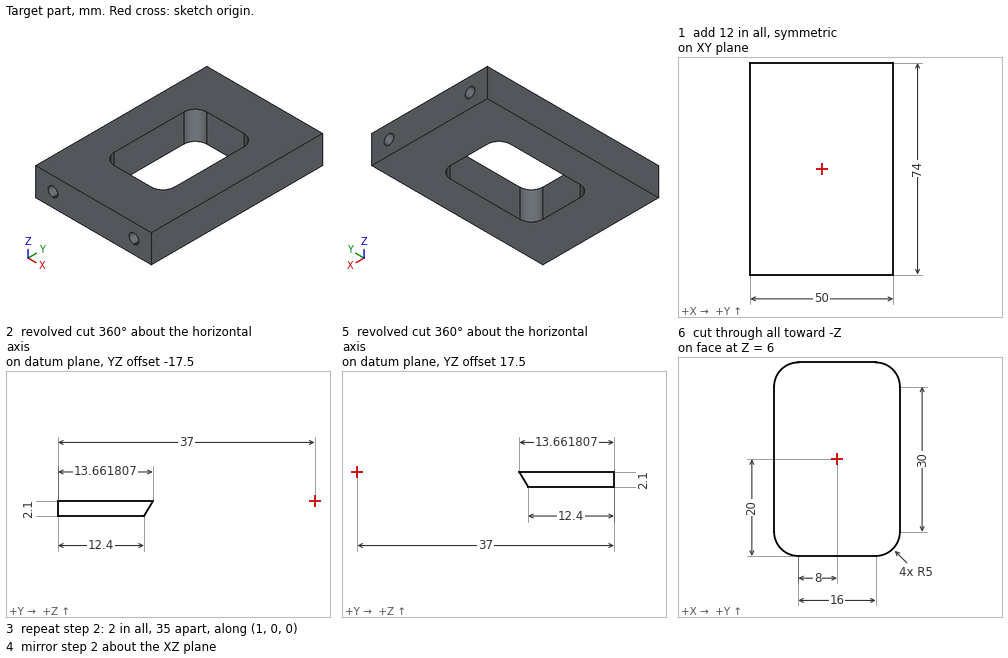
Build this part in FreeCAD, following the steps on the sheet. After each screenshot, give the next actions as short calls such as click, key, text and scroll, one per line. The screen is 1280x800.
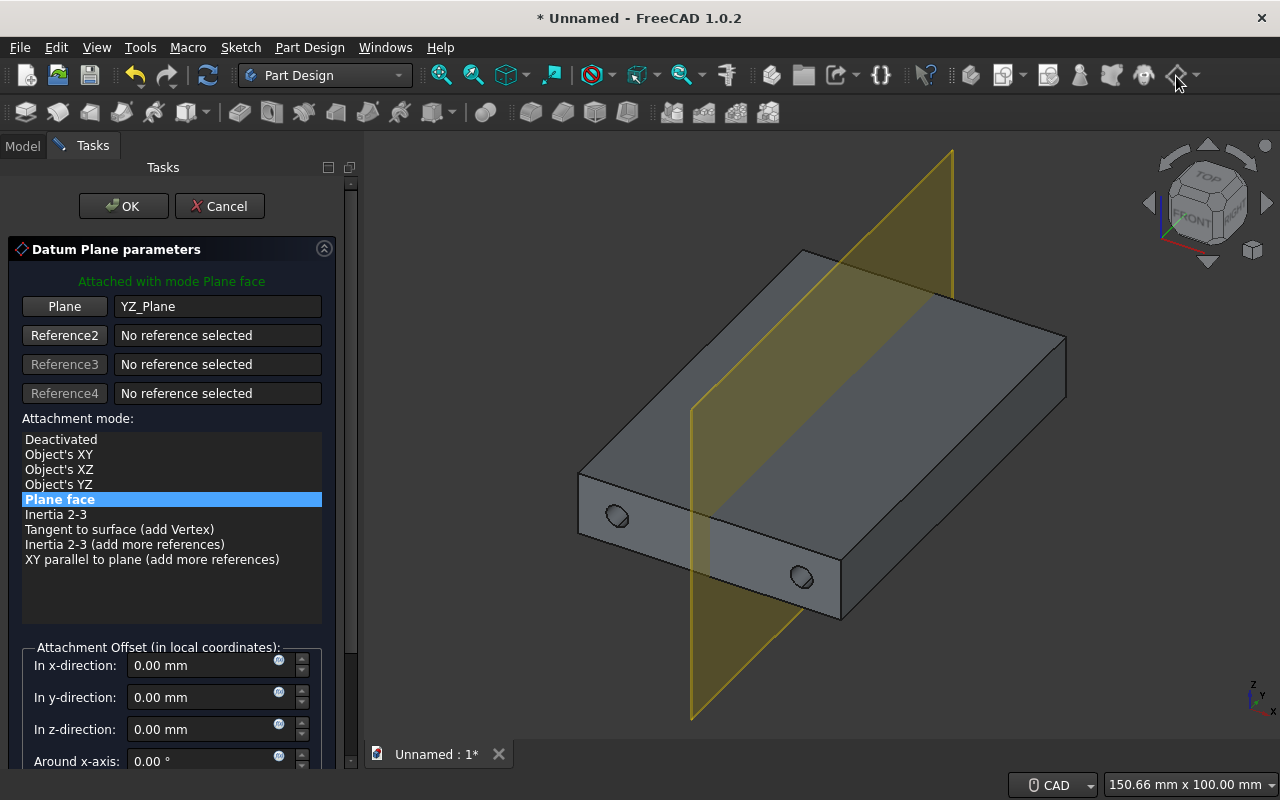
triple_click(210, 729)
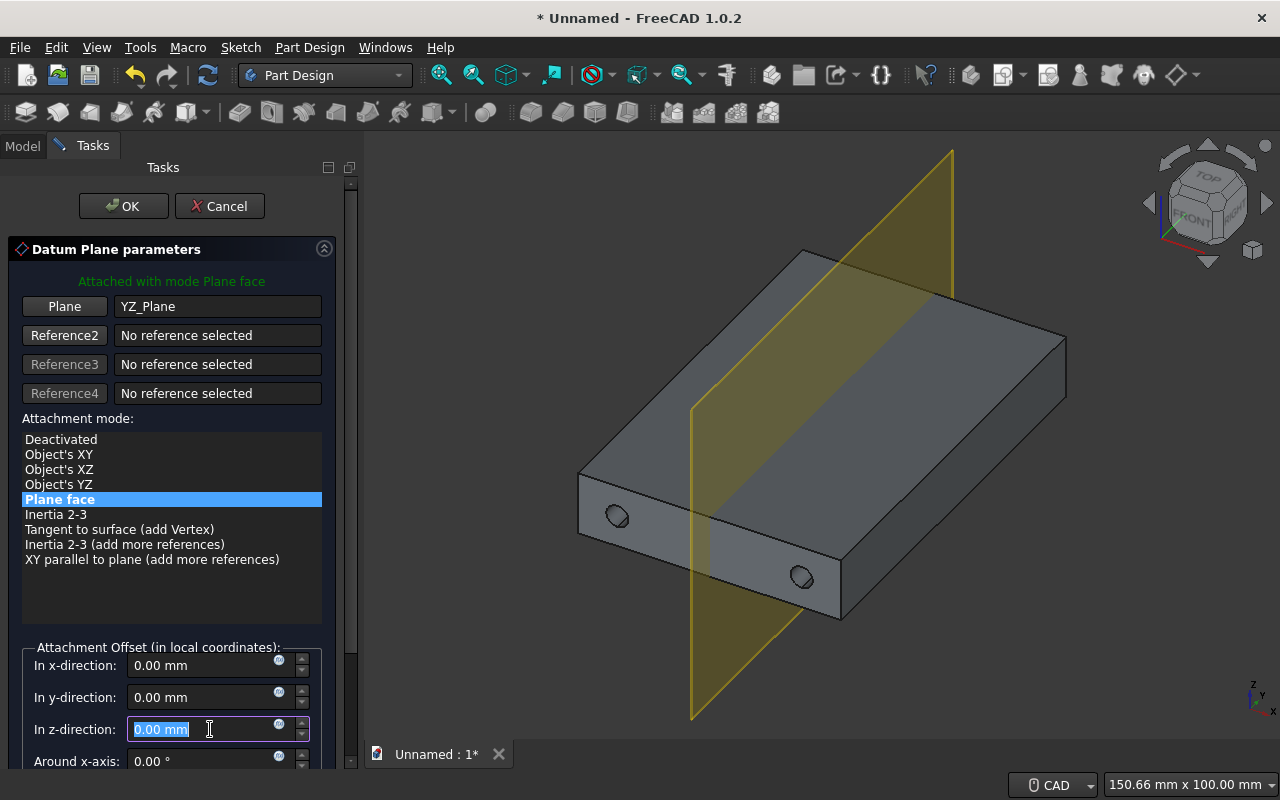
text(17.5)
key(Tab)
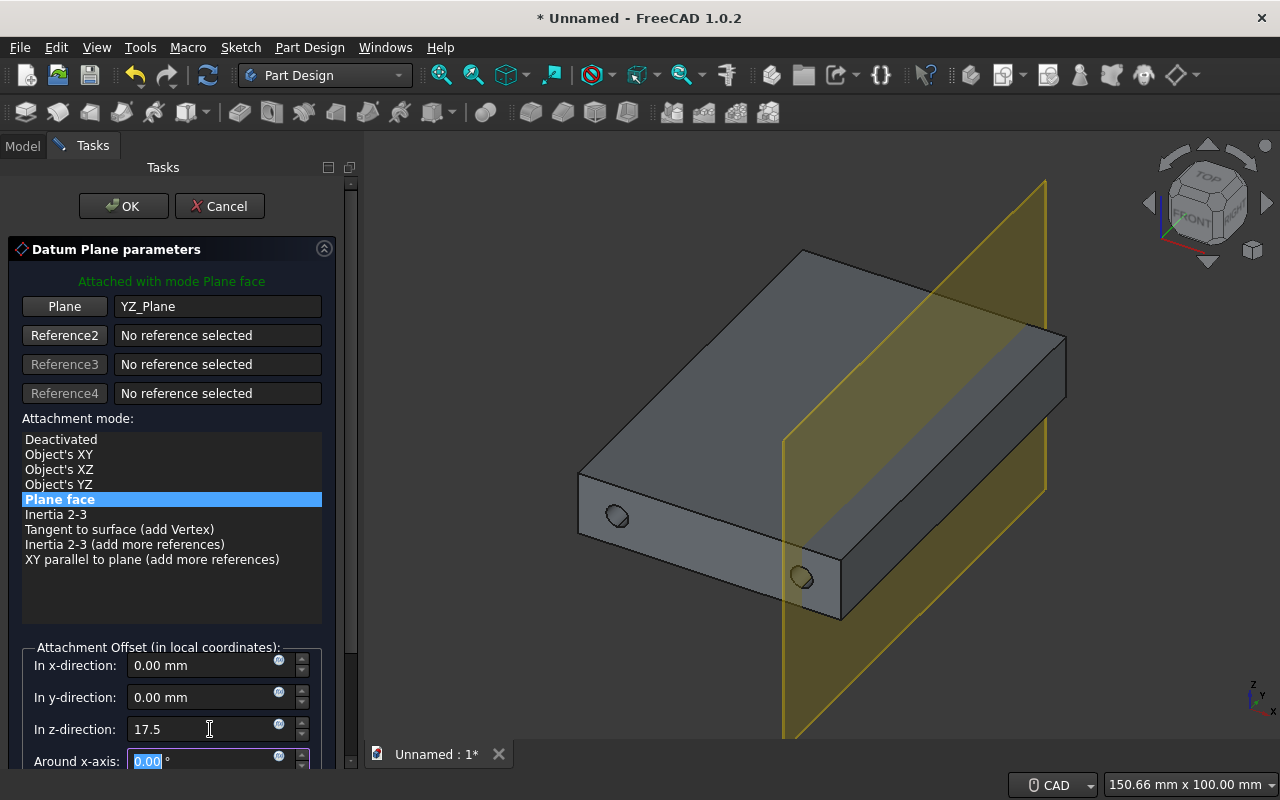
click(124, 206)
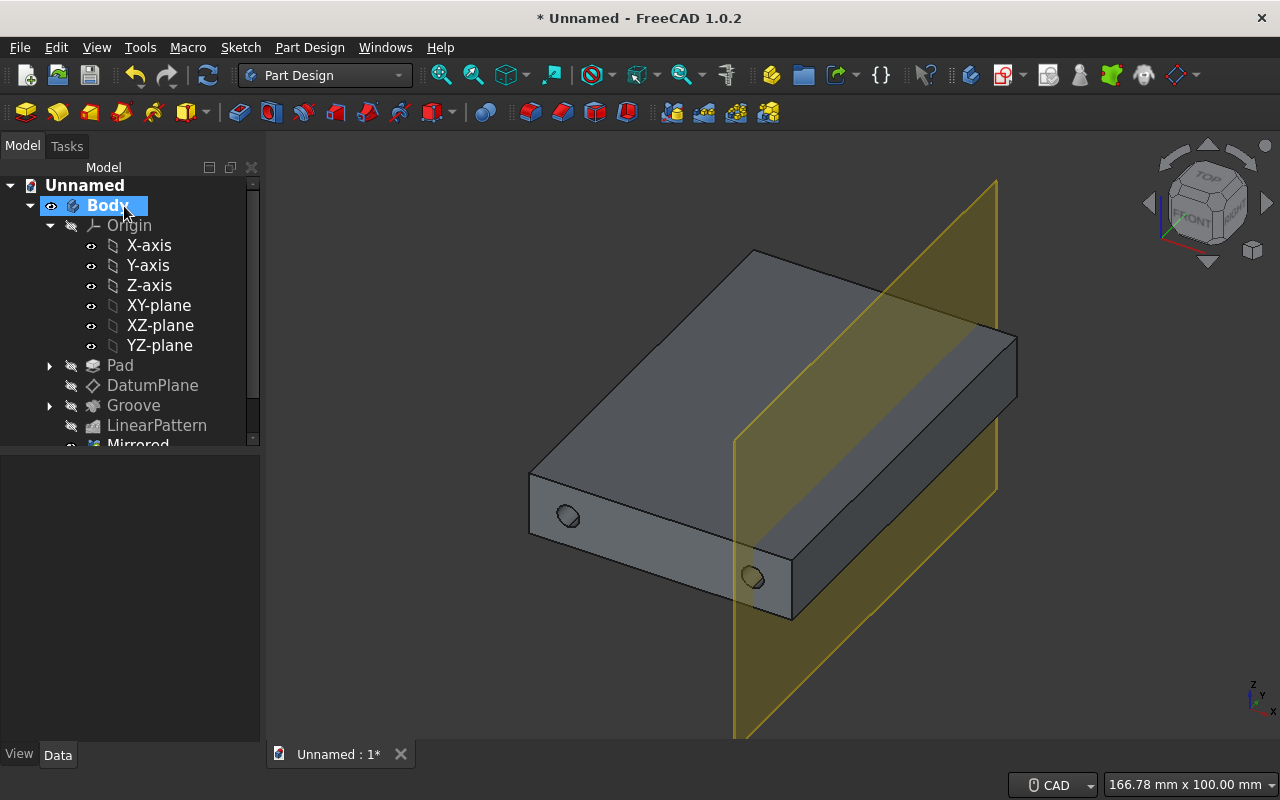
scroll(100, 321, down, 3)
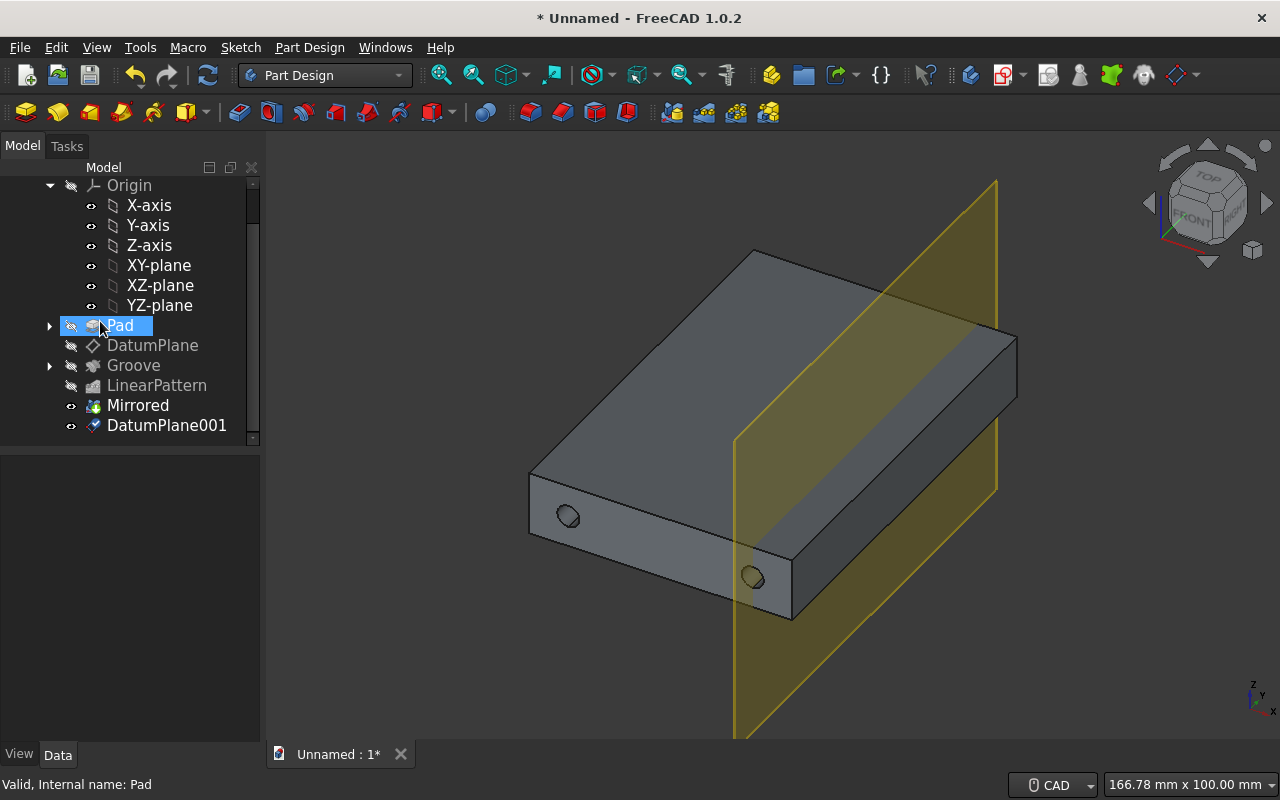
click(116, 426)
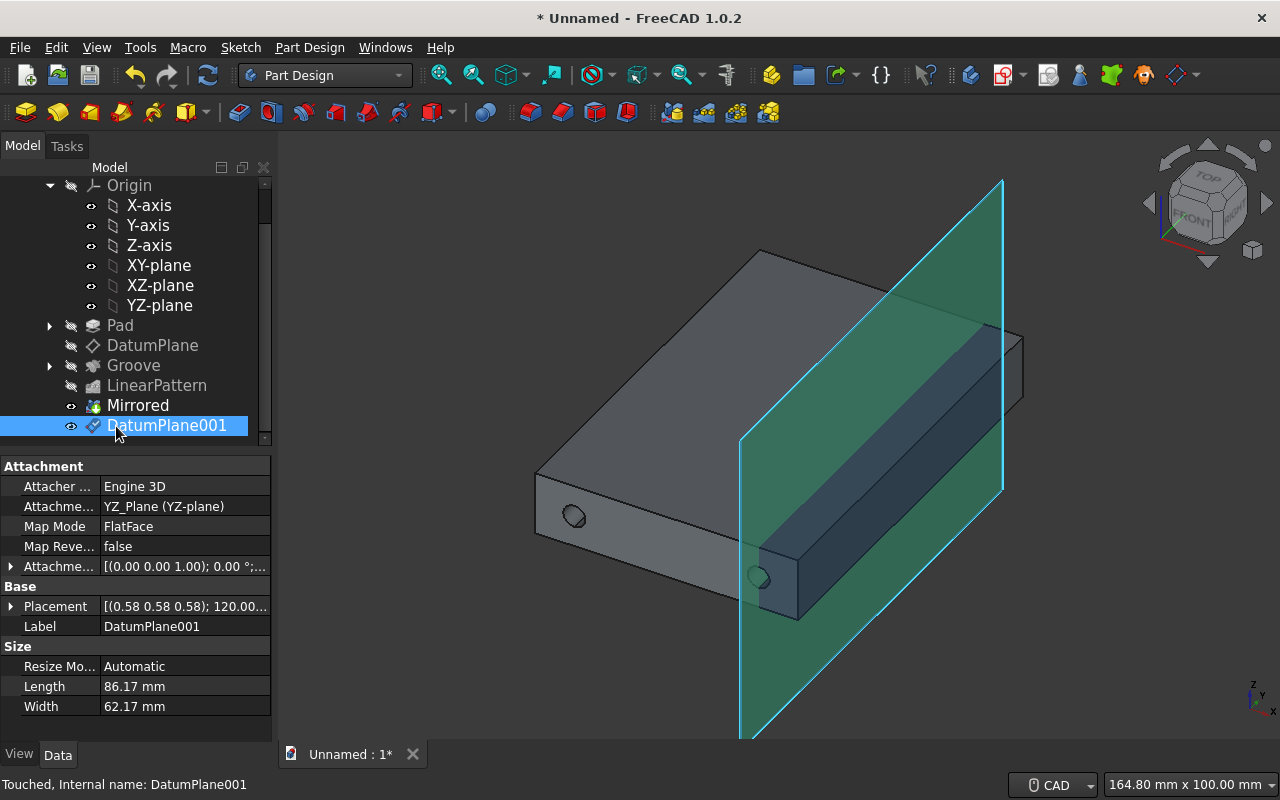
click(1004, 76)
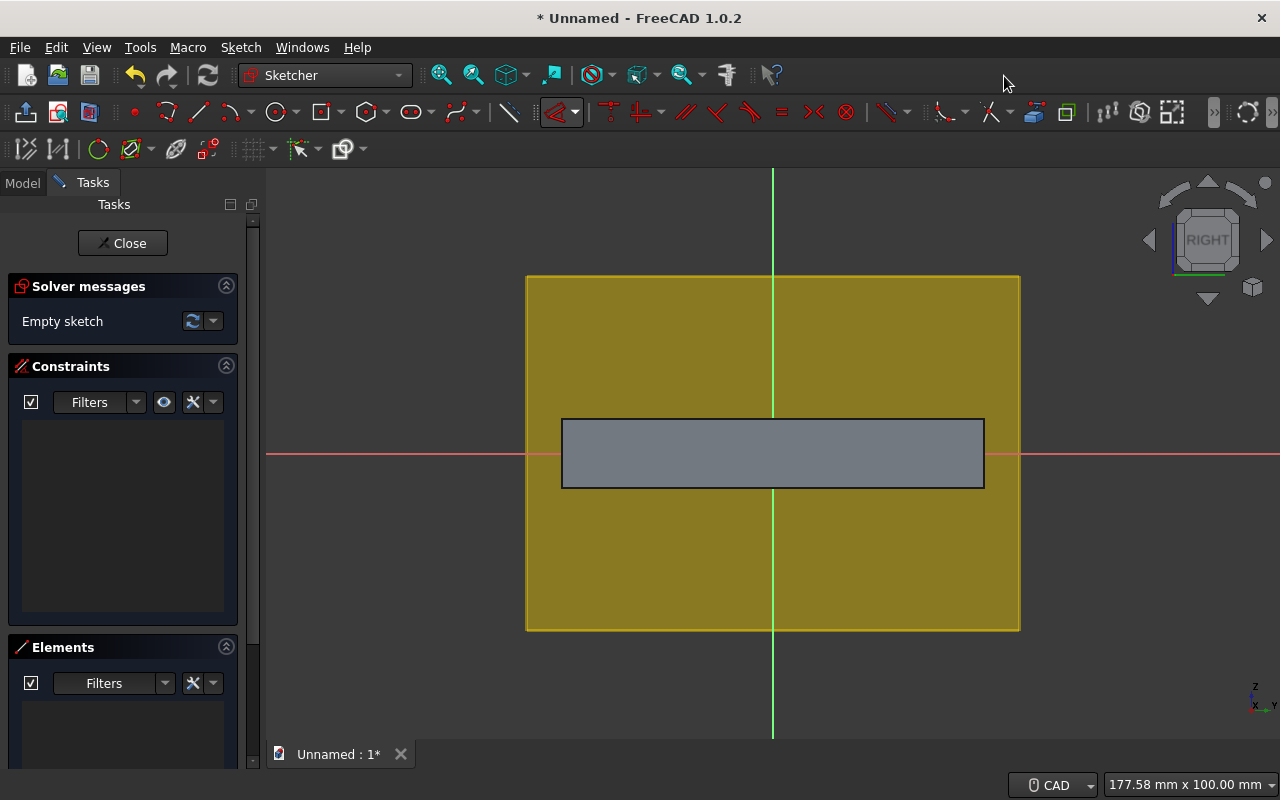
click(90, 112)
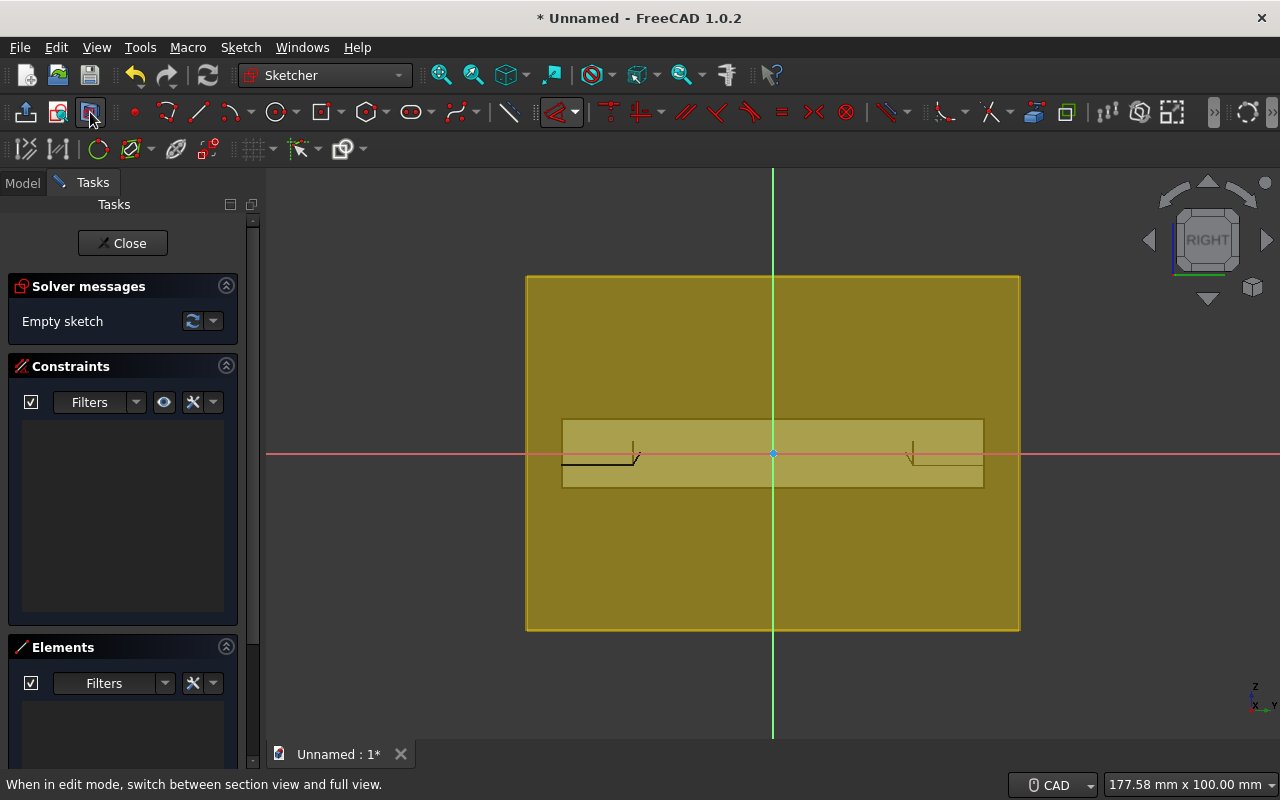
scroll(983, 460, up, 10)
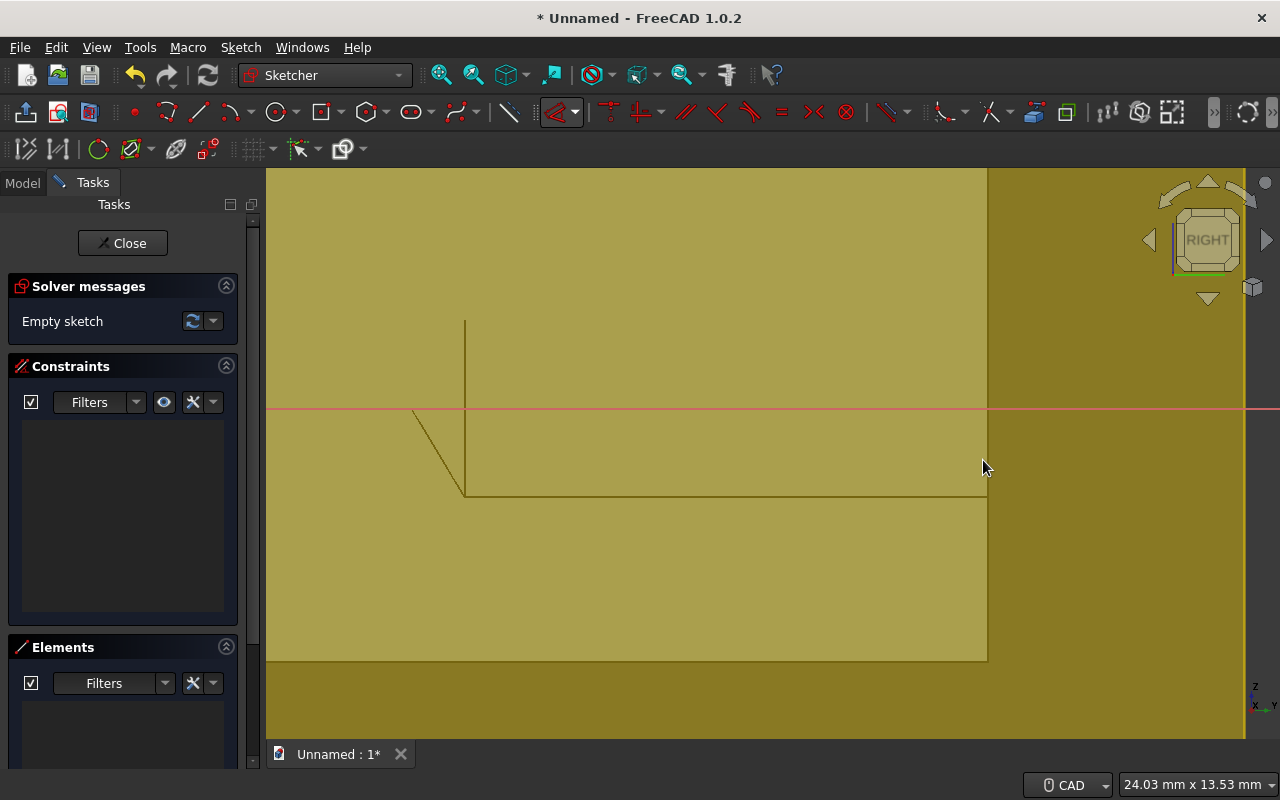
click(168, 112)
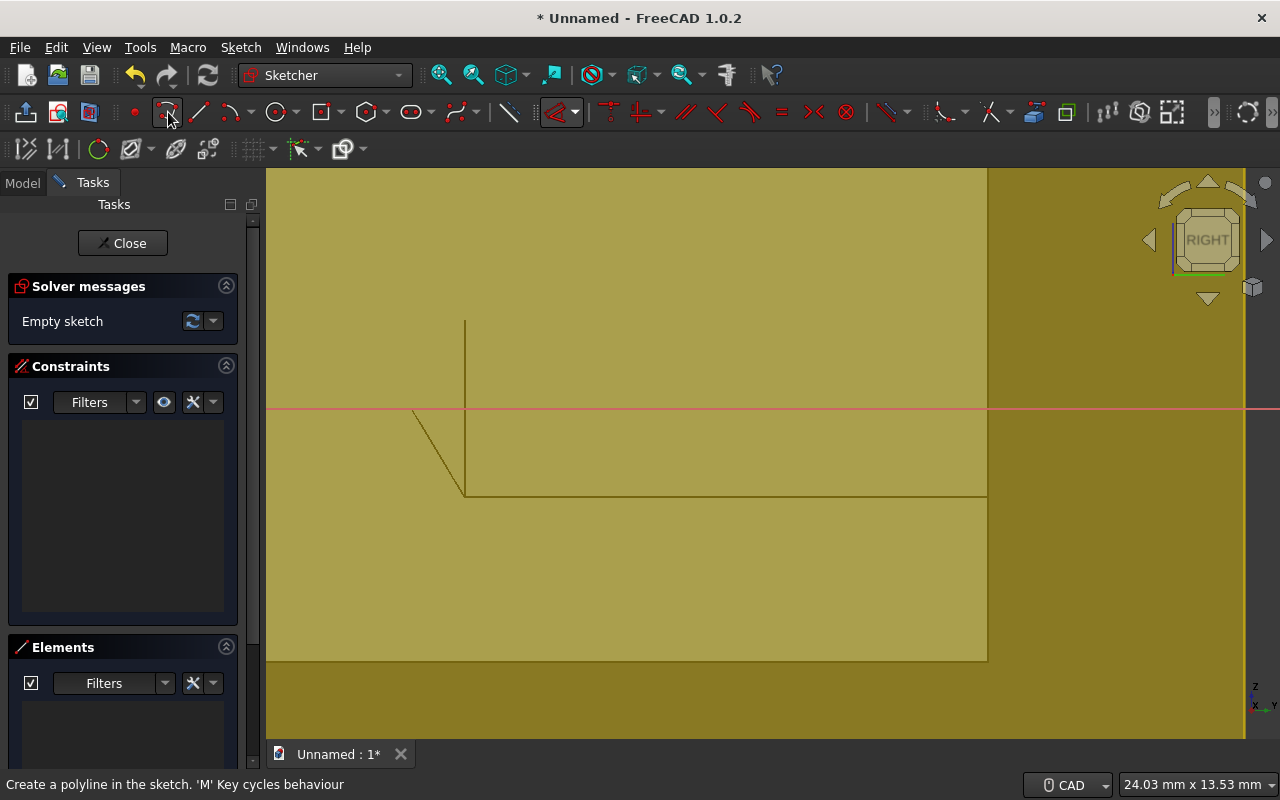
click(411, 409)
click(465, 497)
click(988, 497)
click(988, 418)
click(411, 409)
key(Escape)
key(Escape)